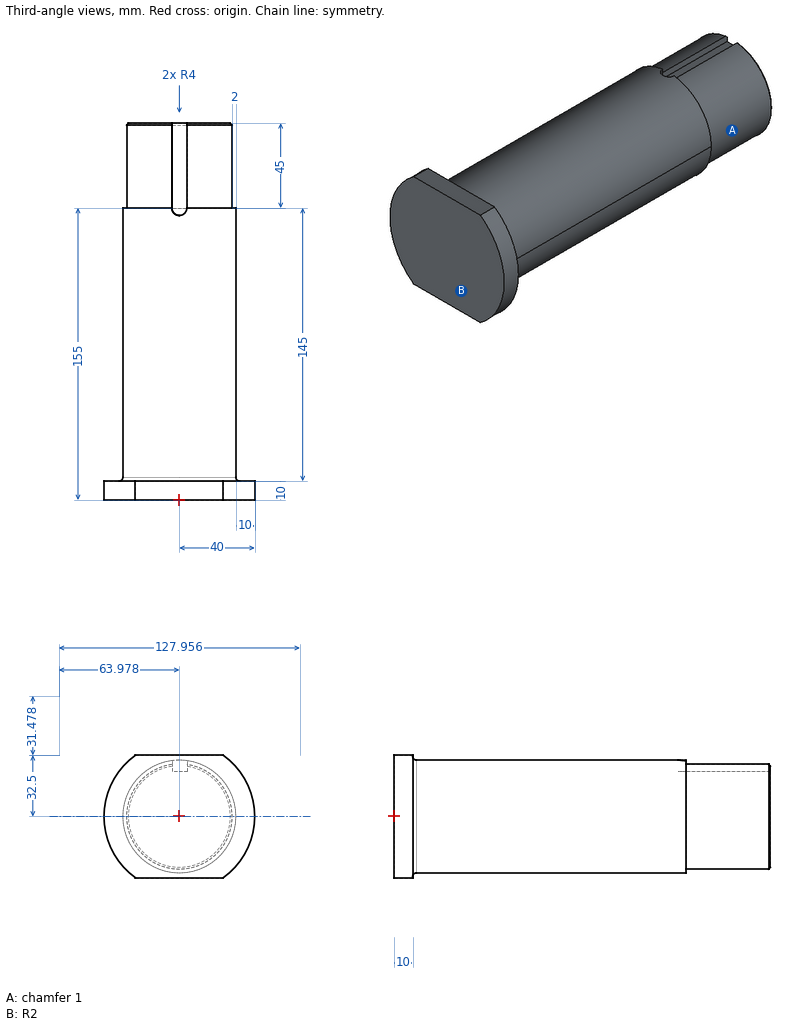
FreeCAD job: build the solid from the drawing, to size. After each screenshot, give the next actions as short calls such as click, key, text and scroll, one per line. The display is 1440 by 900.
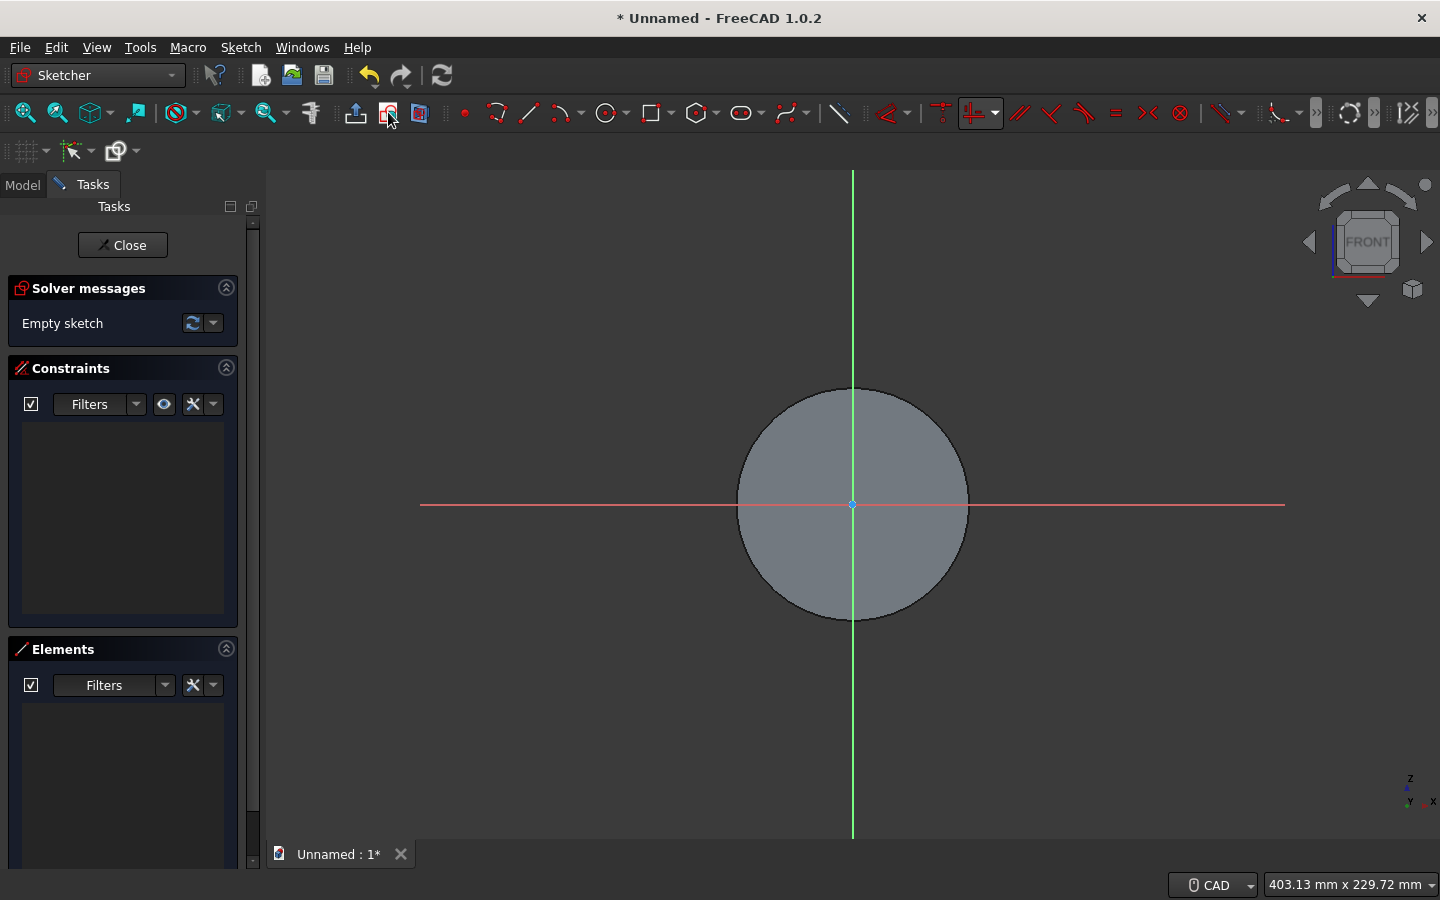
click(652, 114)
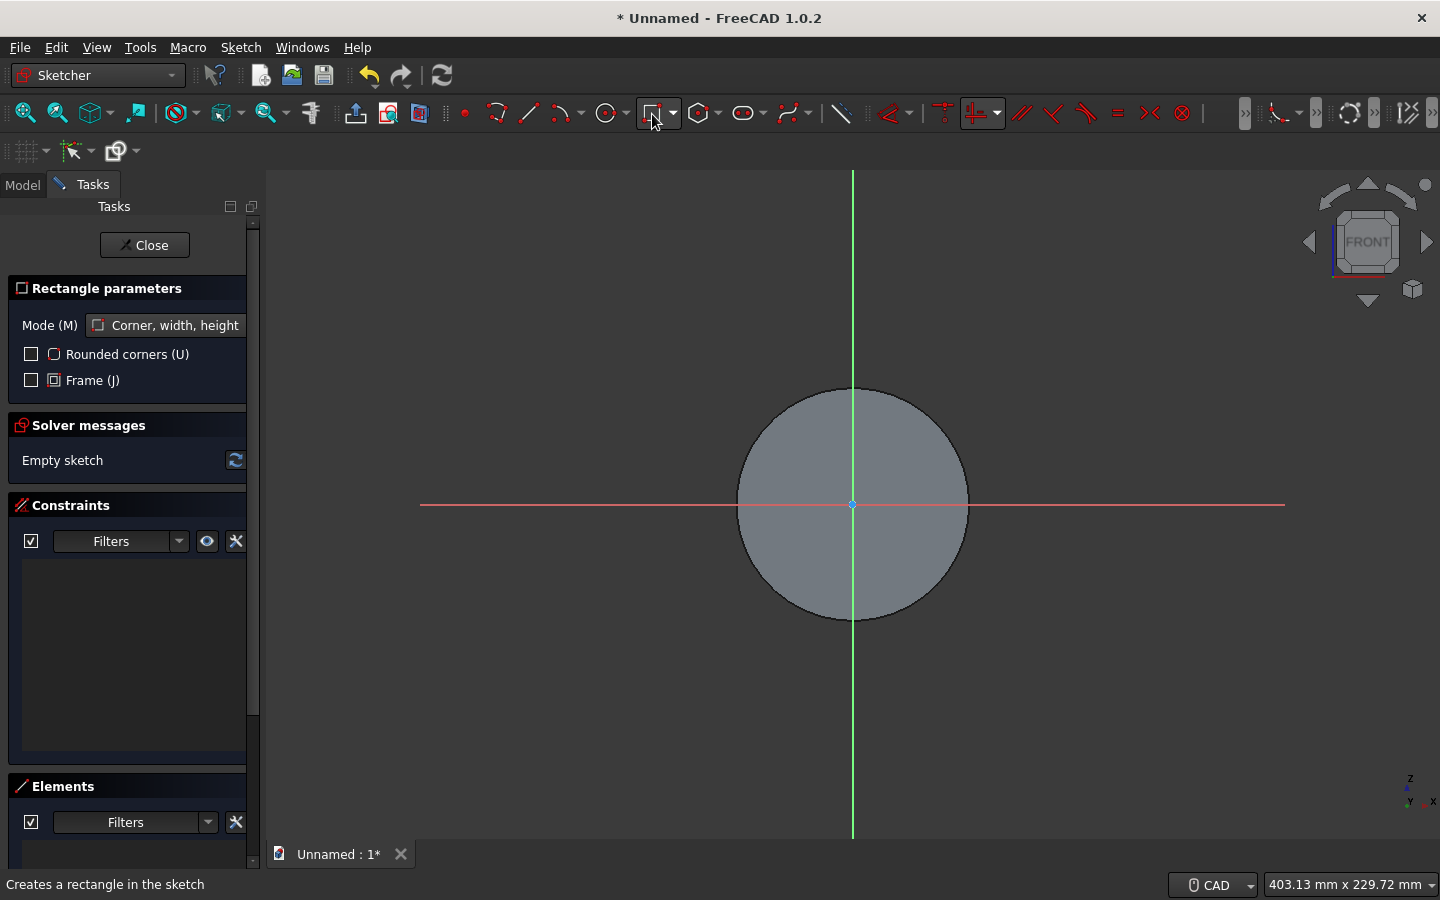
click(667, 318)
click(1039, 410)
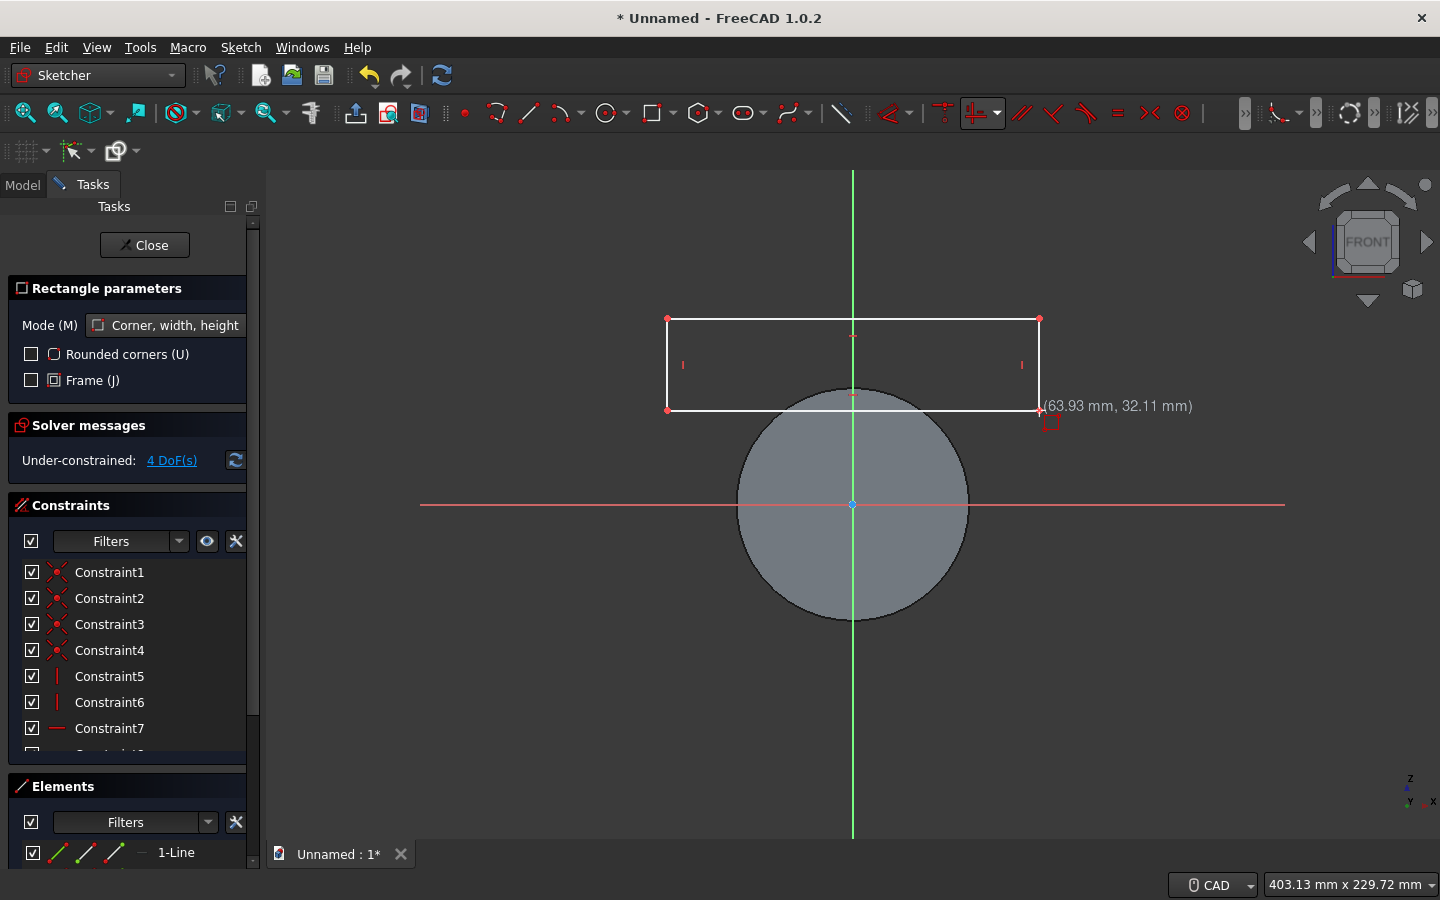
click(667, 599)
click(1039, 691)
key(Escape)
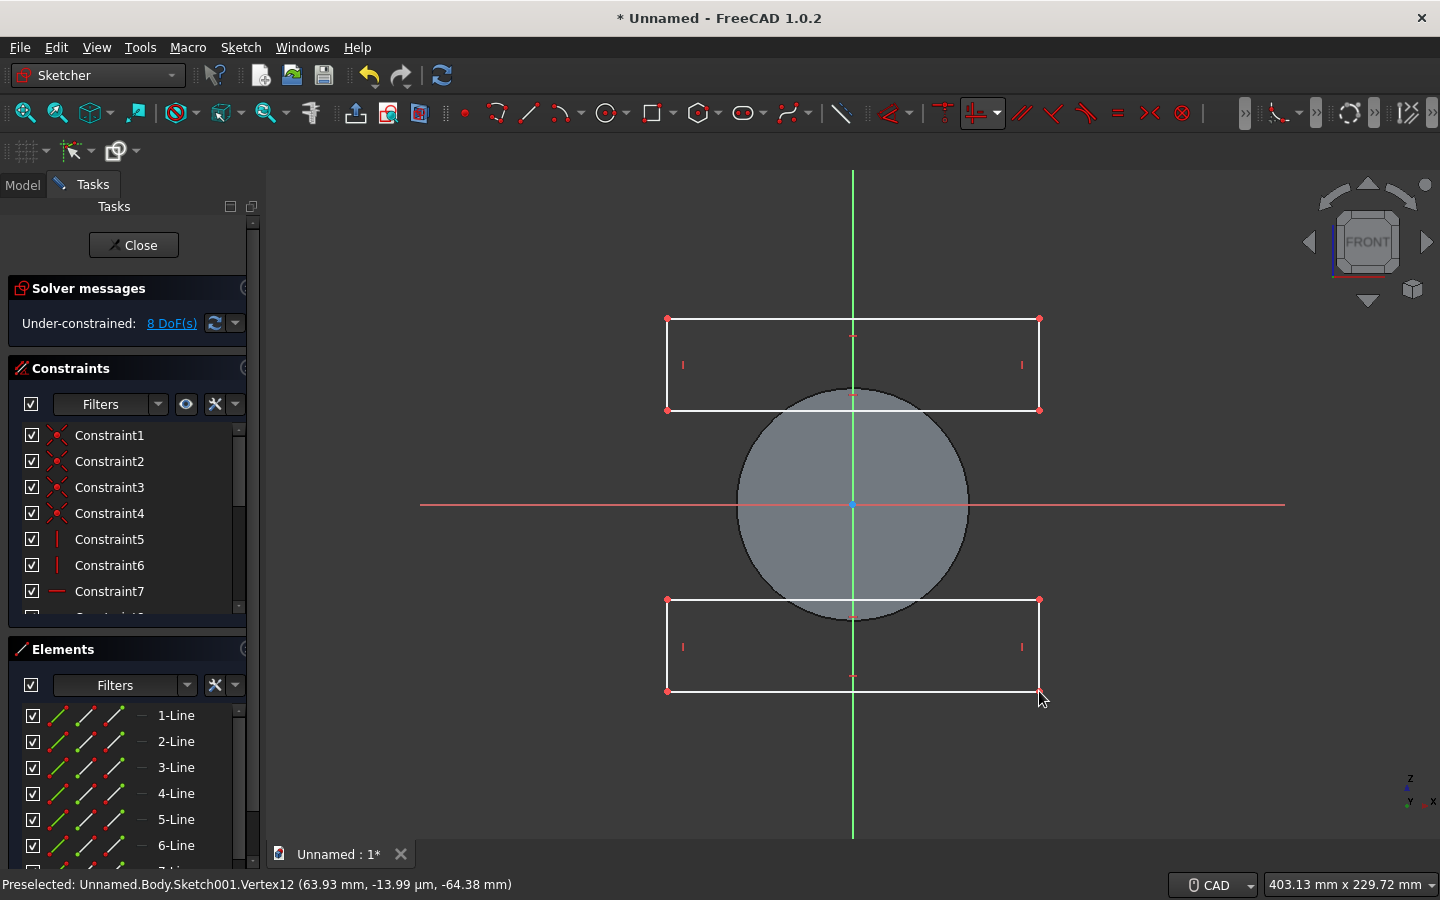
click(667, 411)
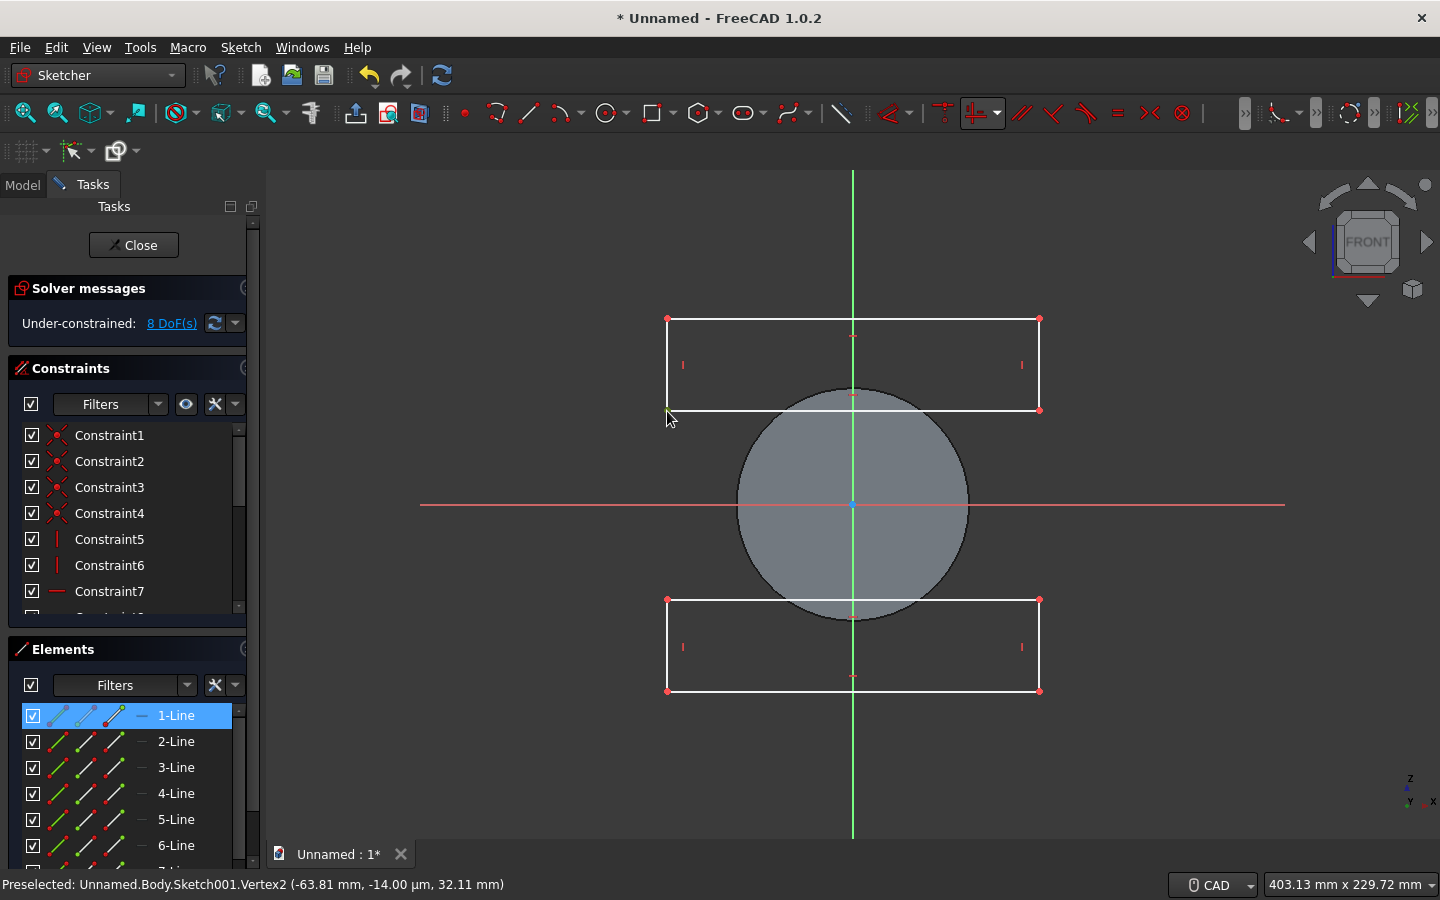
click(667, 600)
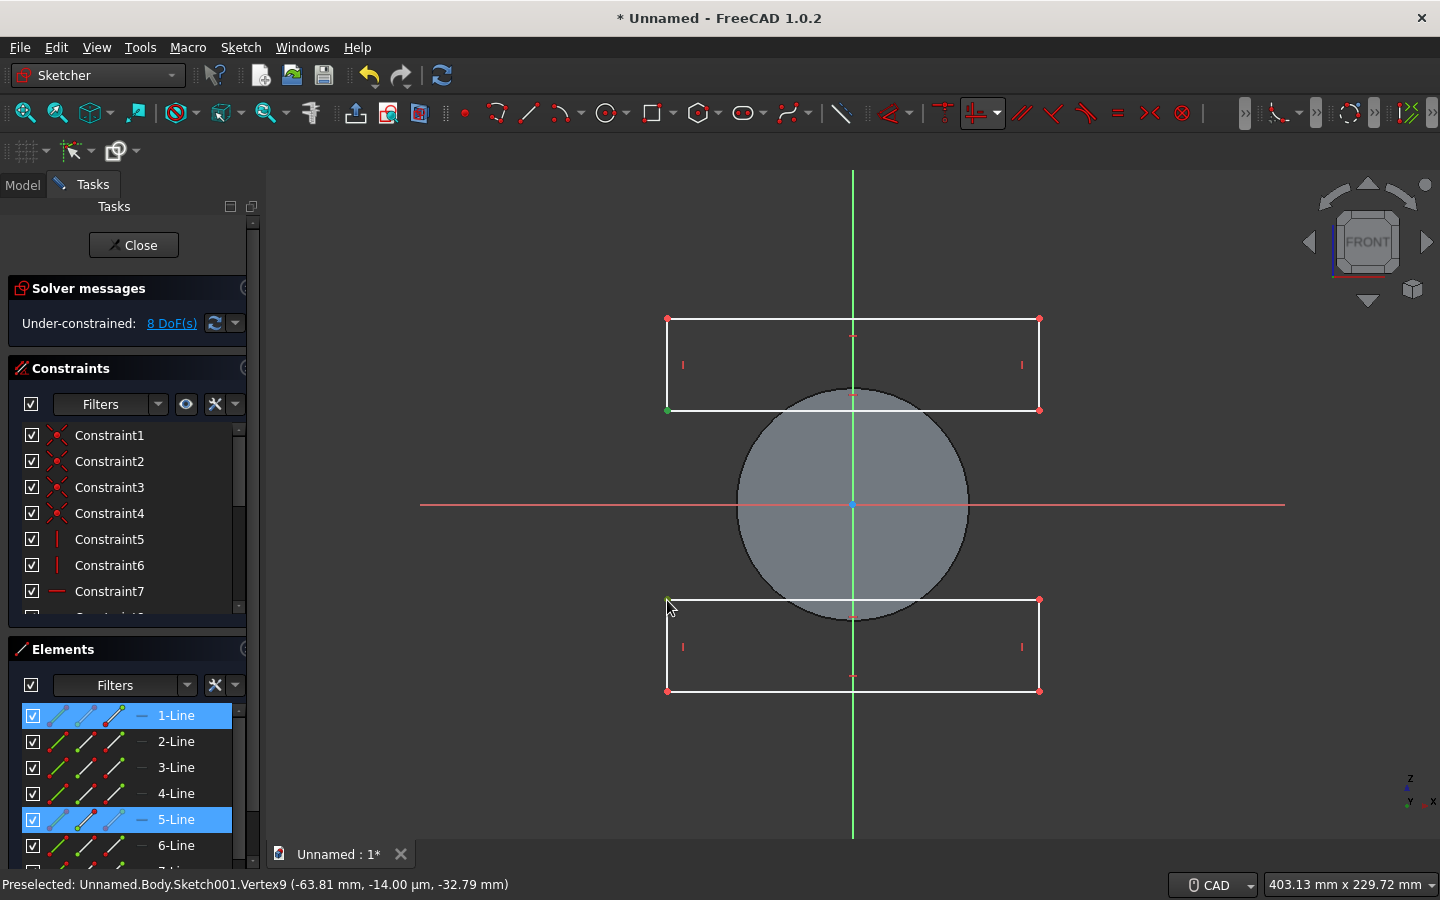
click(434, 505)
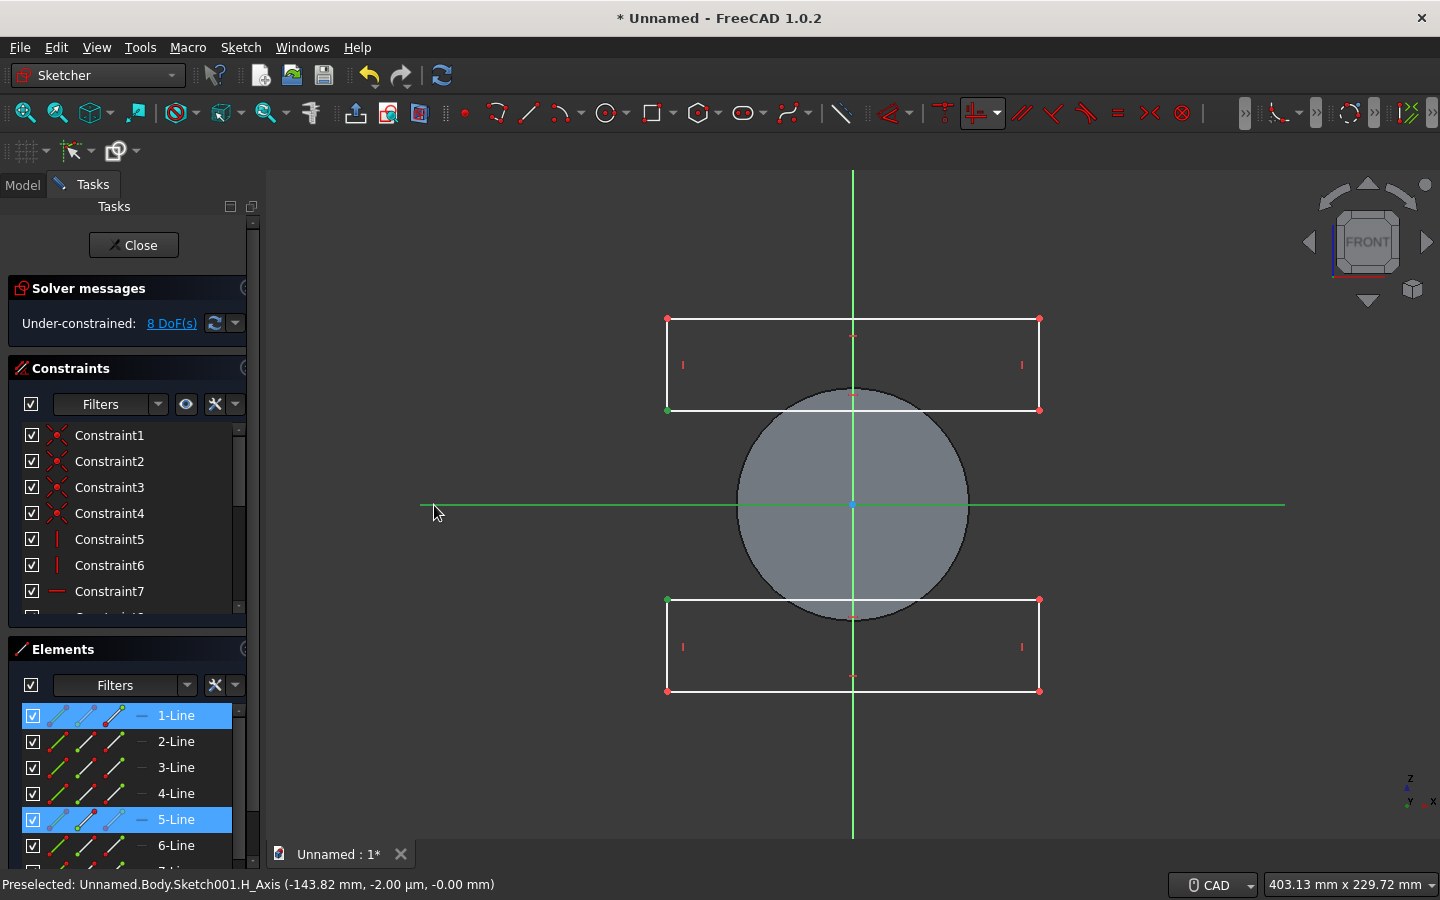
click(1150, 114)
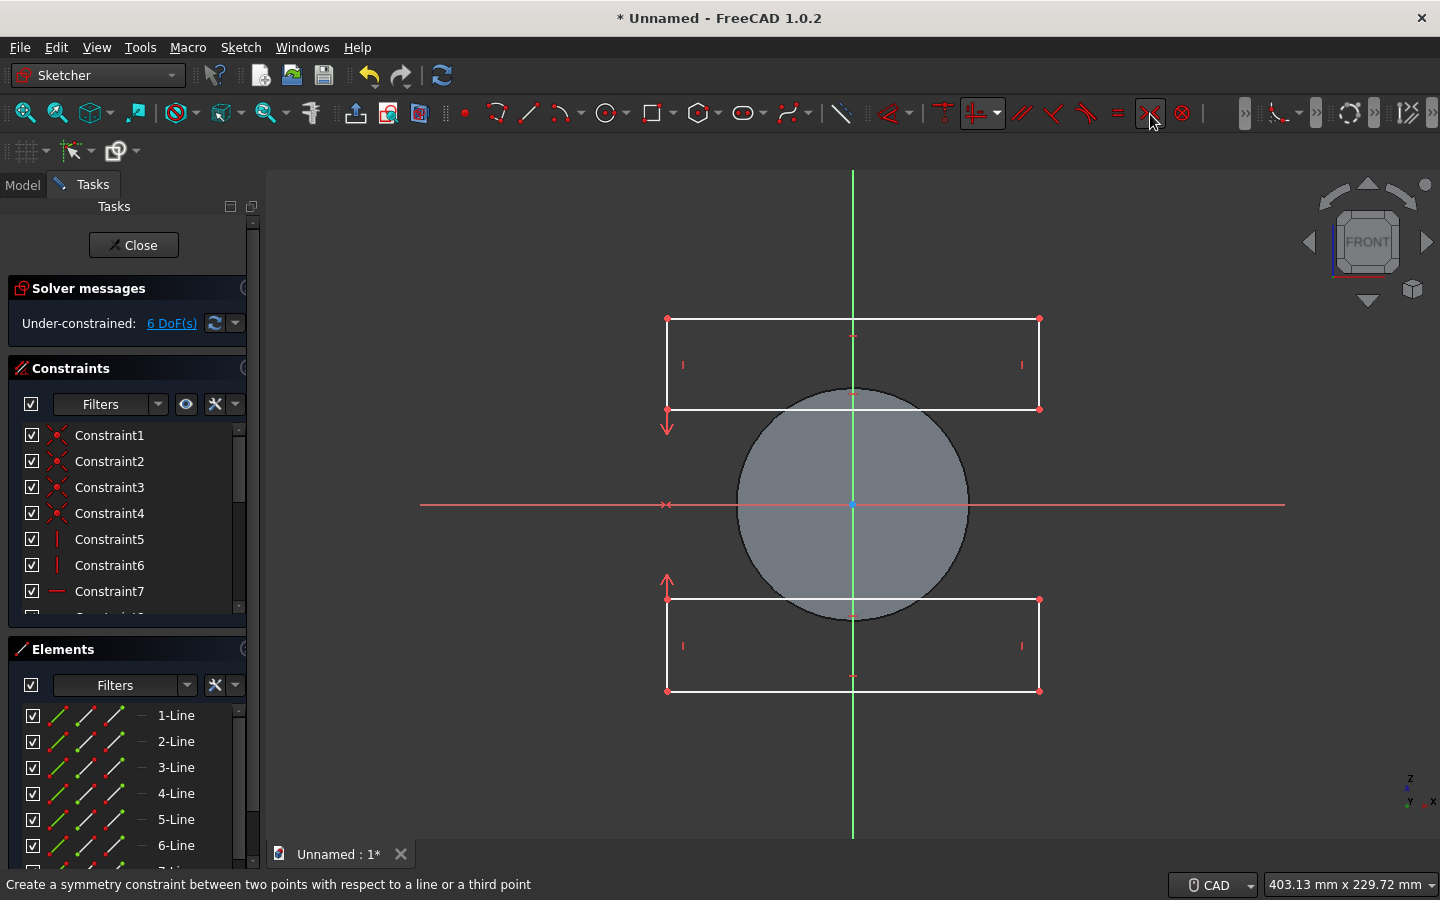
click(1039, 319)